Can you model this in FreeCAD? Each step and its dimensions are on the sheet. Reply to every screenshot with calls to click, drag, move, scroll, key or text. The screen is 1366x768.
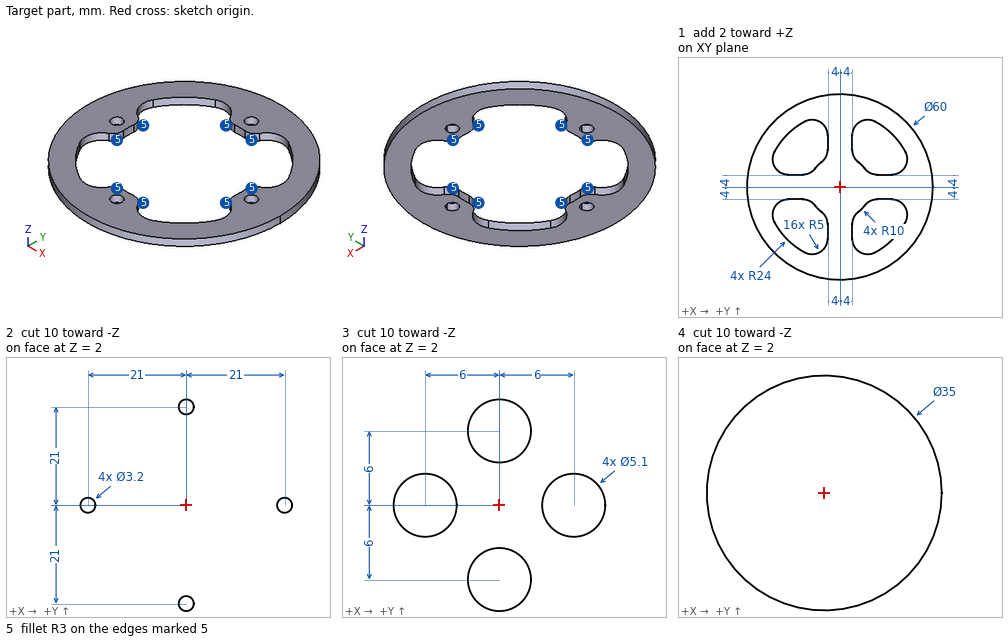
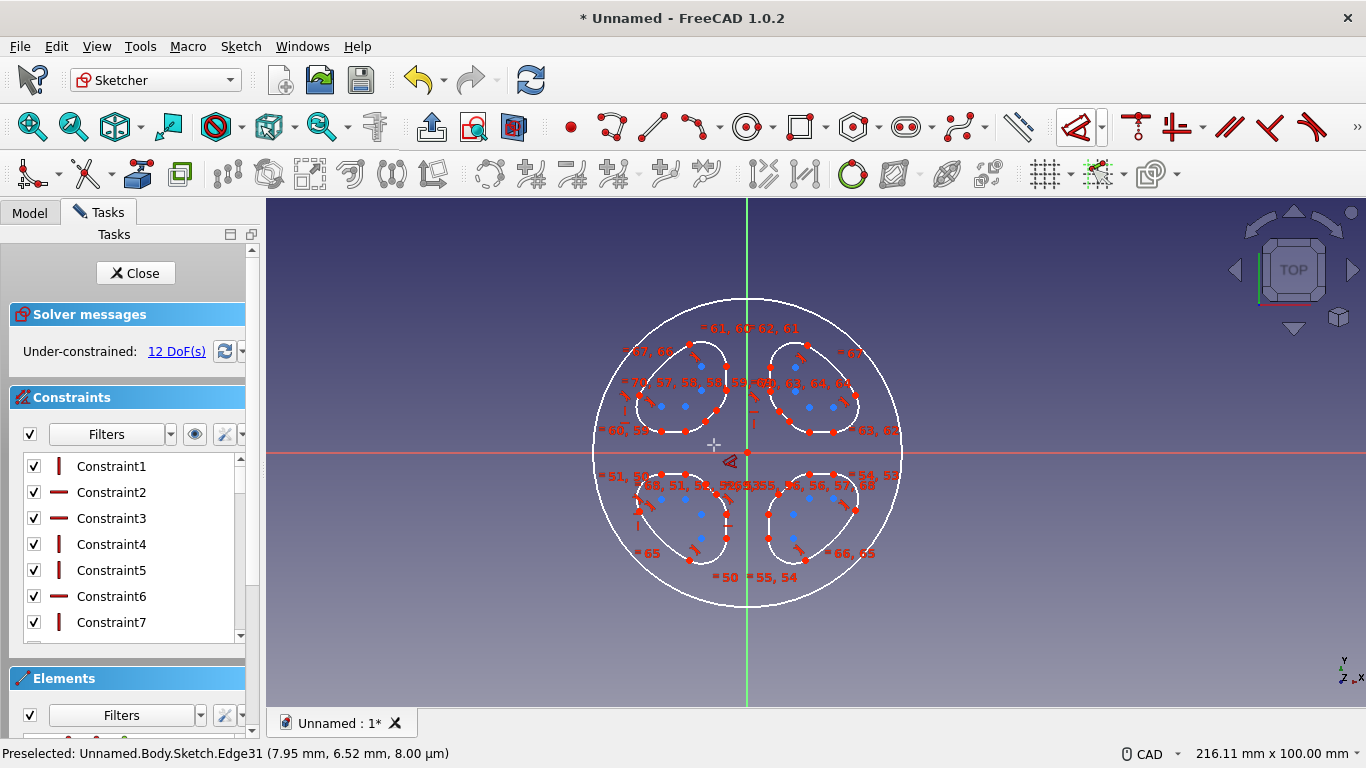
scroll(705, 563, up, 3)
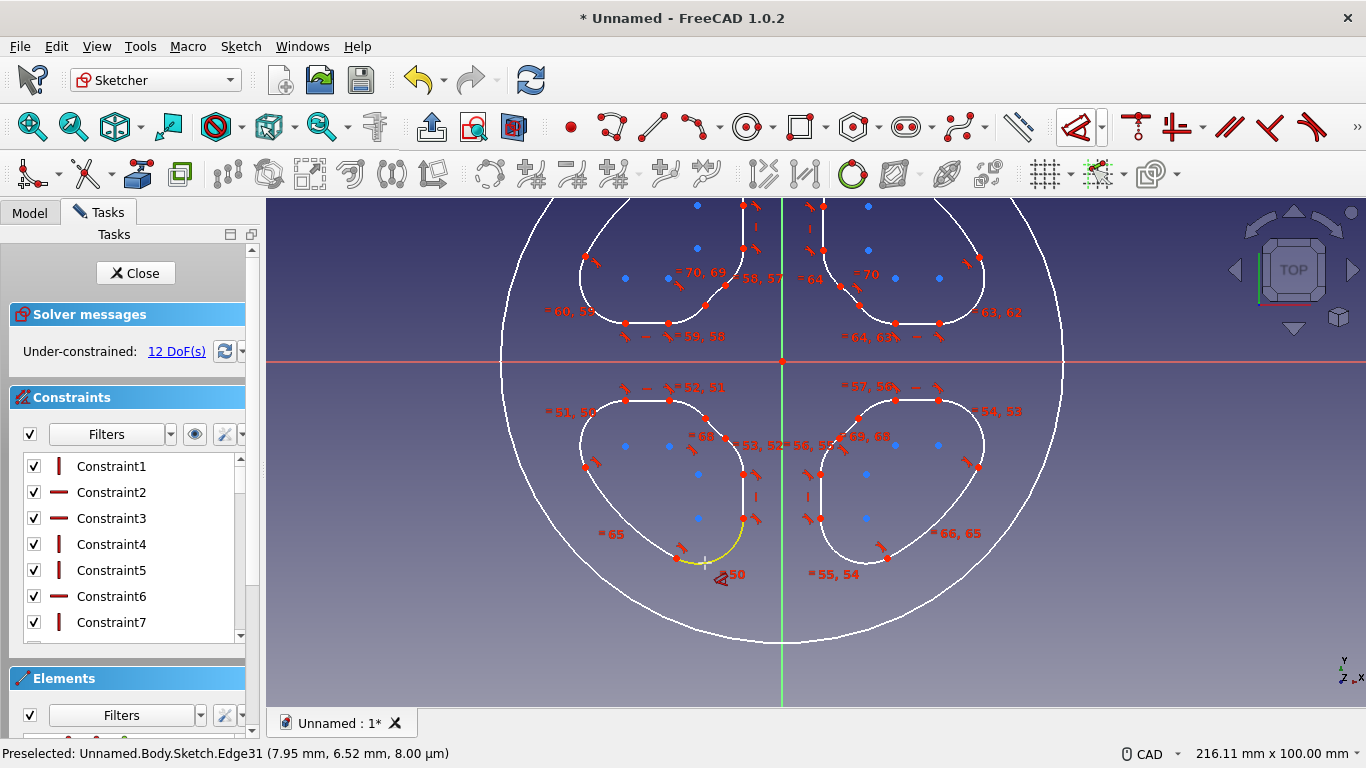
click(704, 563)
click(708, 595)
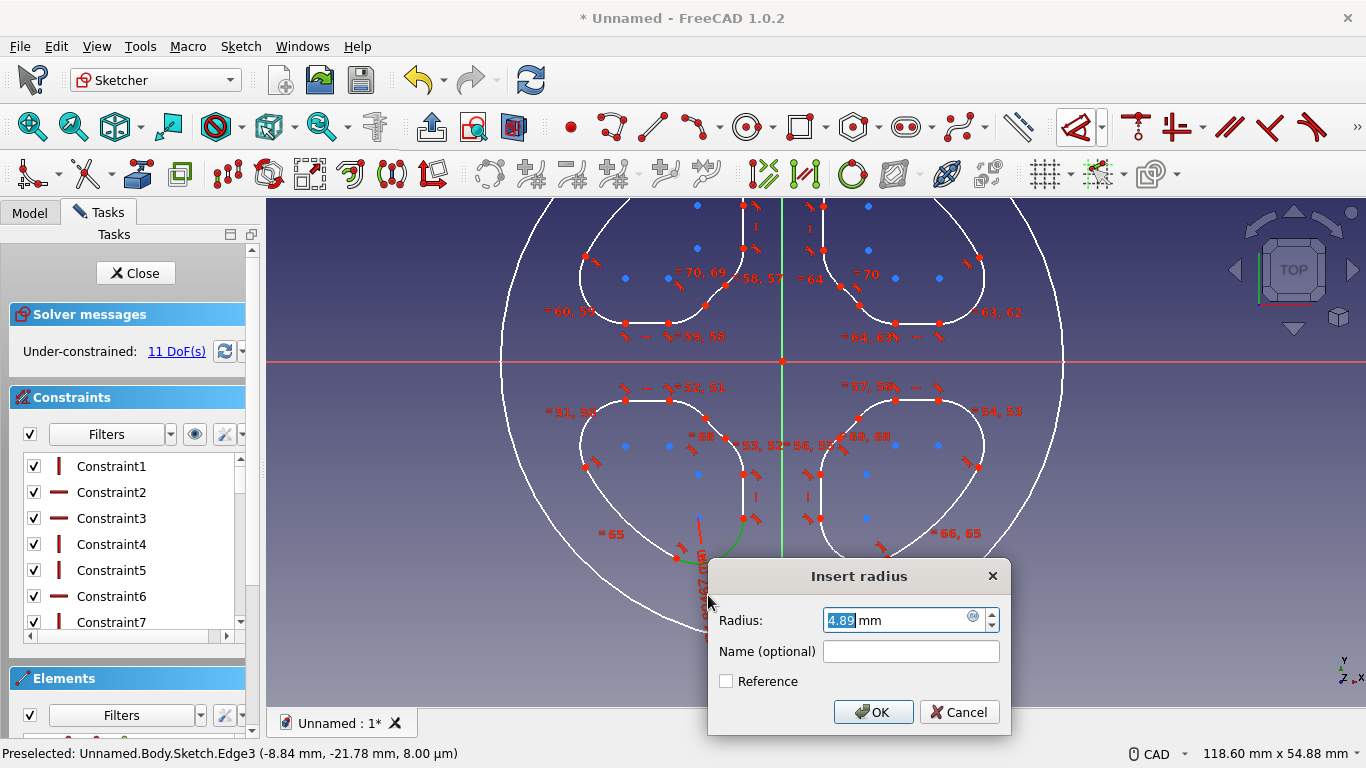
text(5)
key(Return)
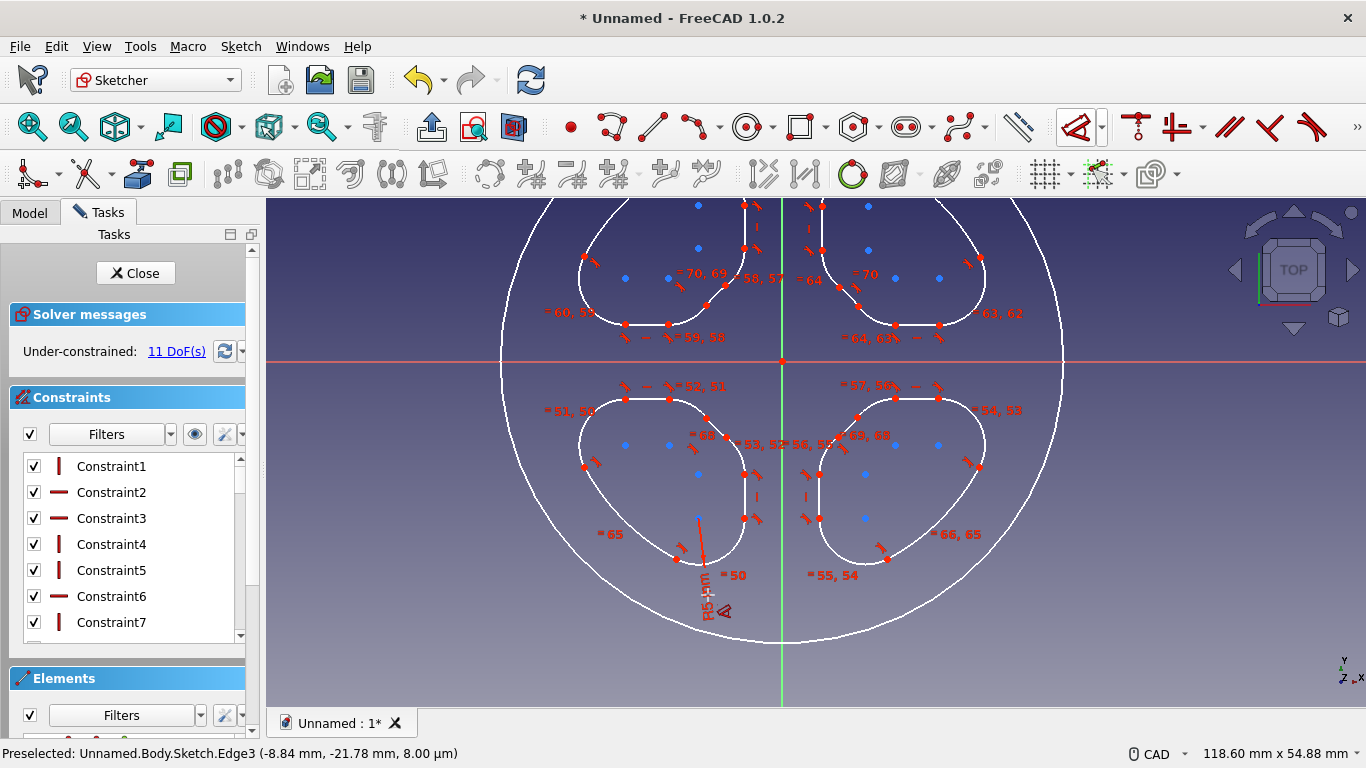
click(607, 501)
click(582, 521)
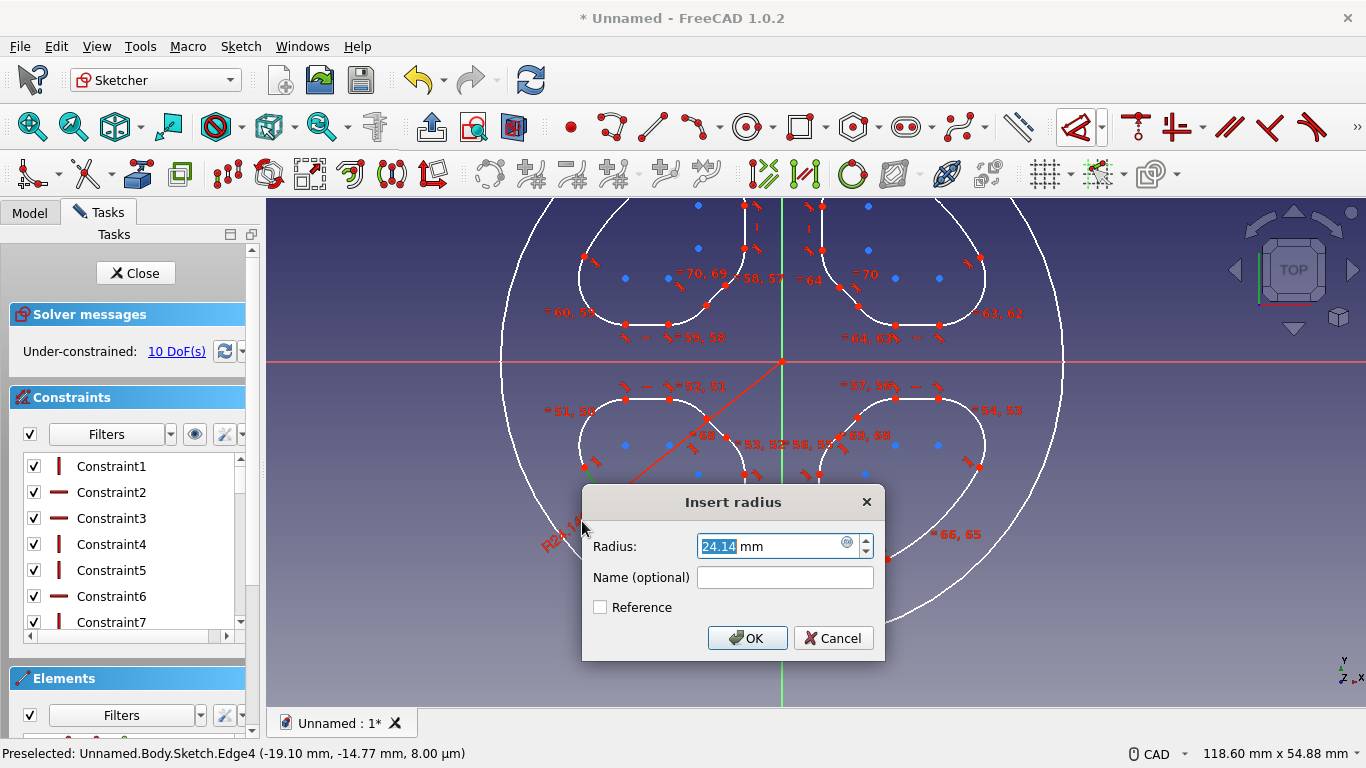
text(24)
key(Return)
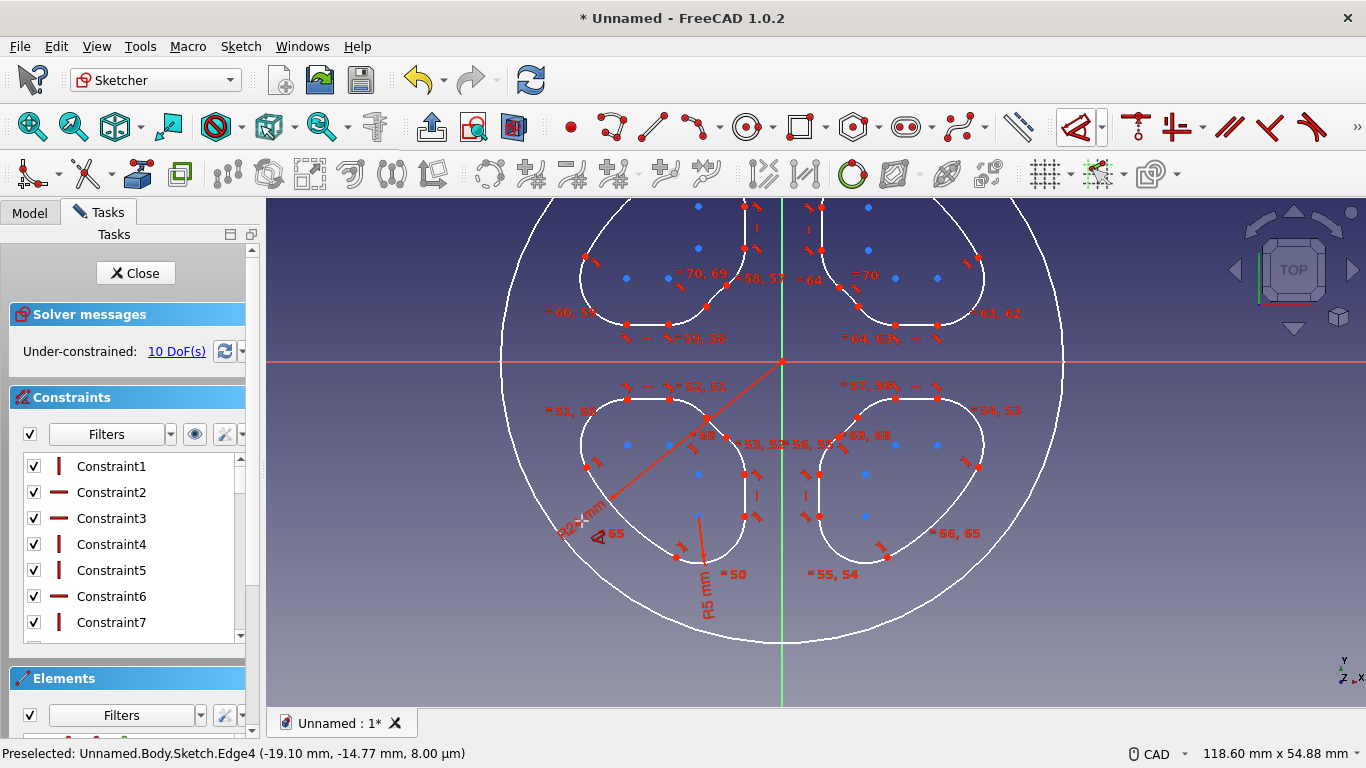
click(716, 428)
click(693, 451)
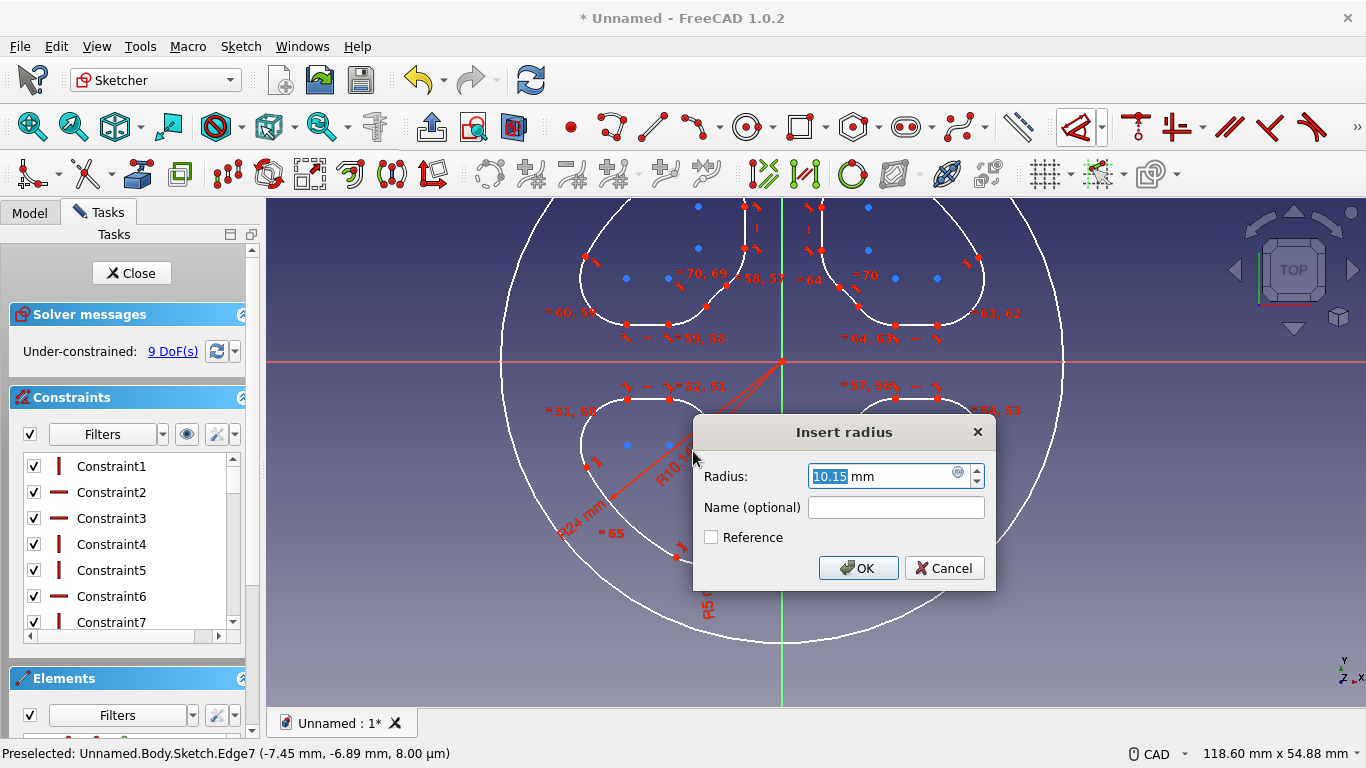
text(10)
key(Return)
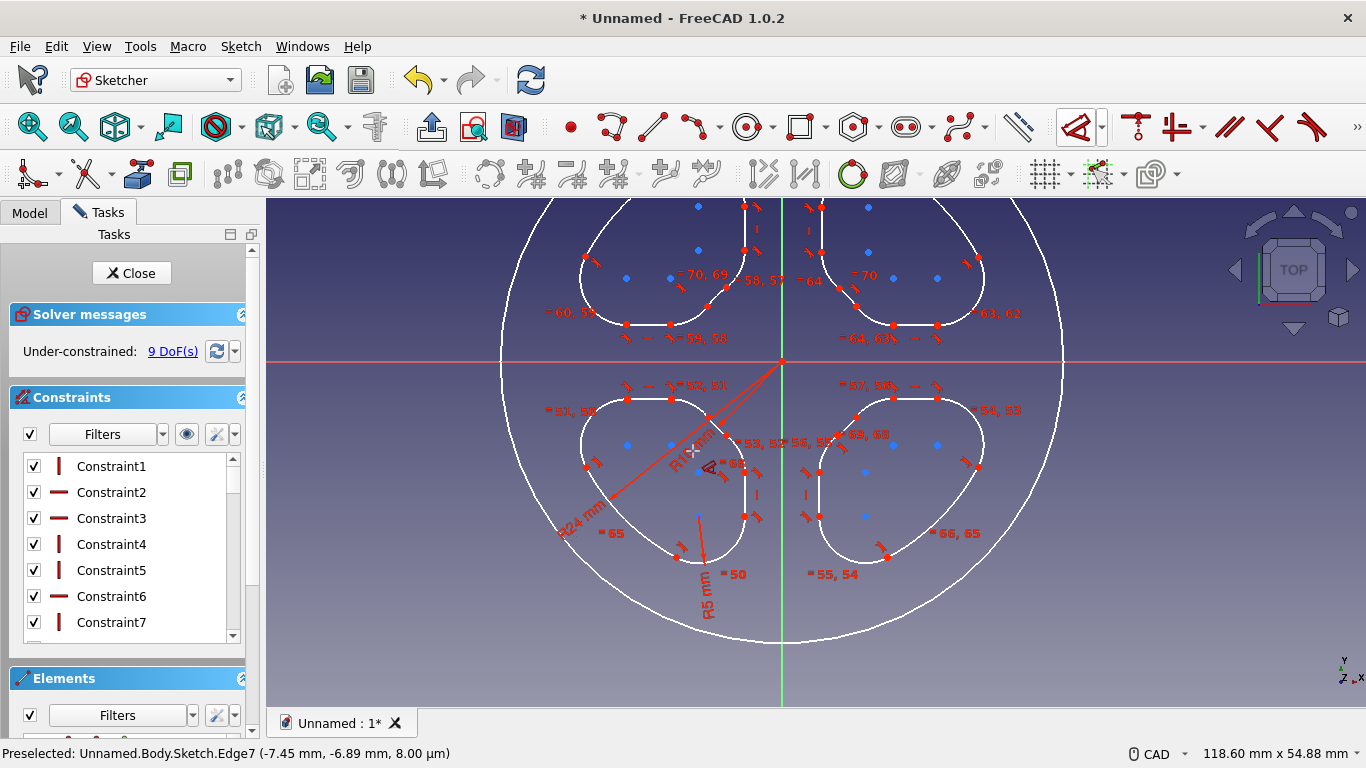
click(584, 561)
click(561, 584)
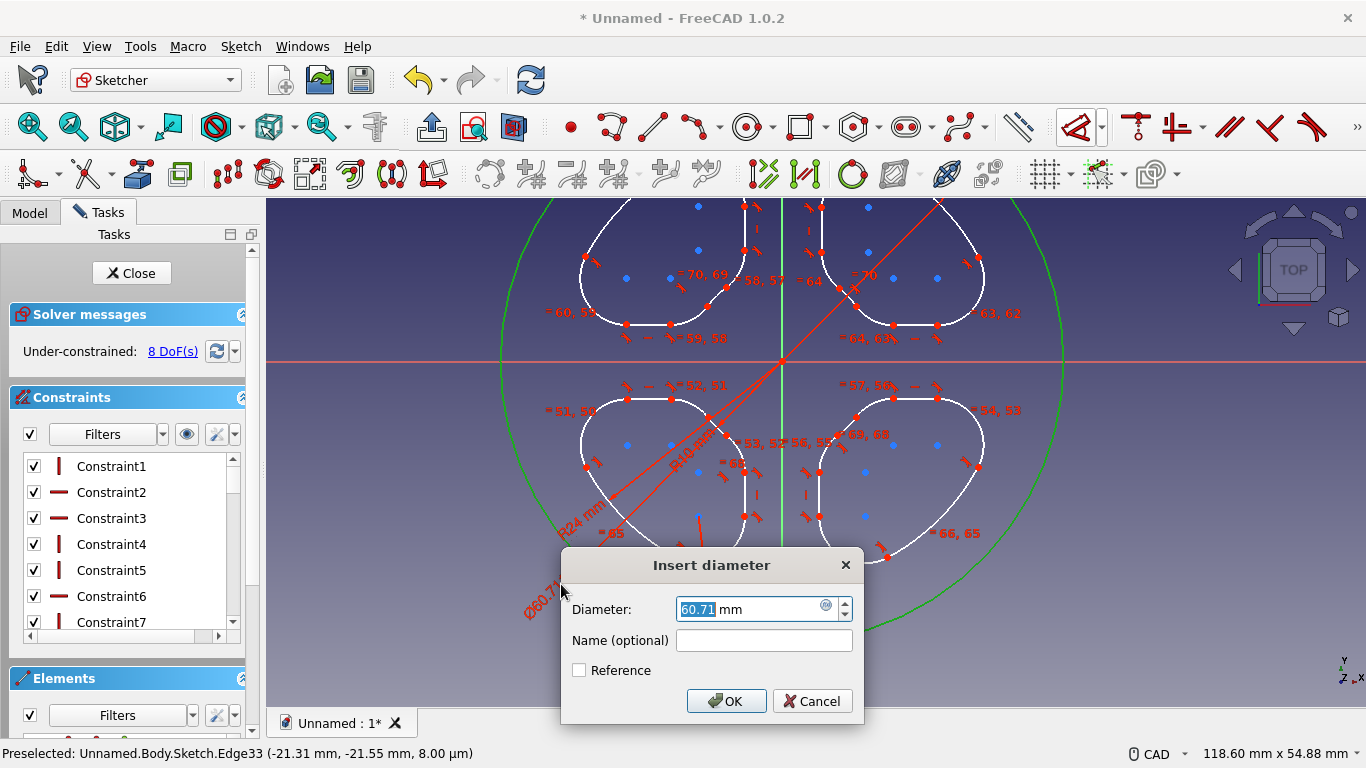
text(60)
key(Return)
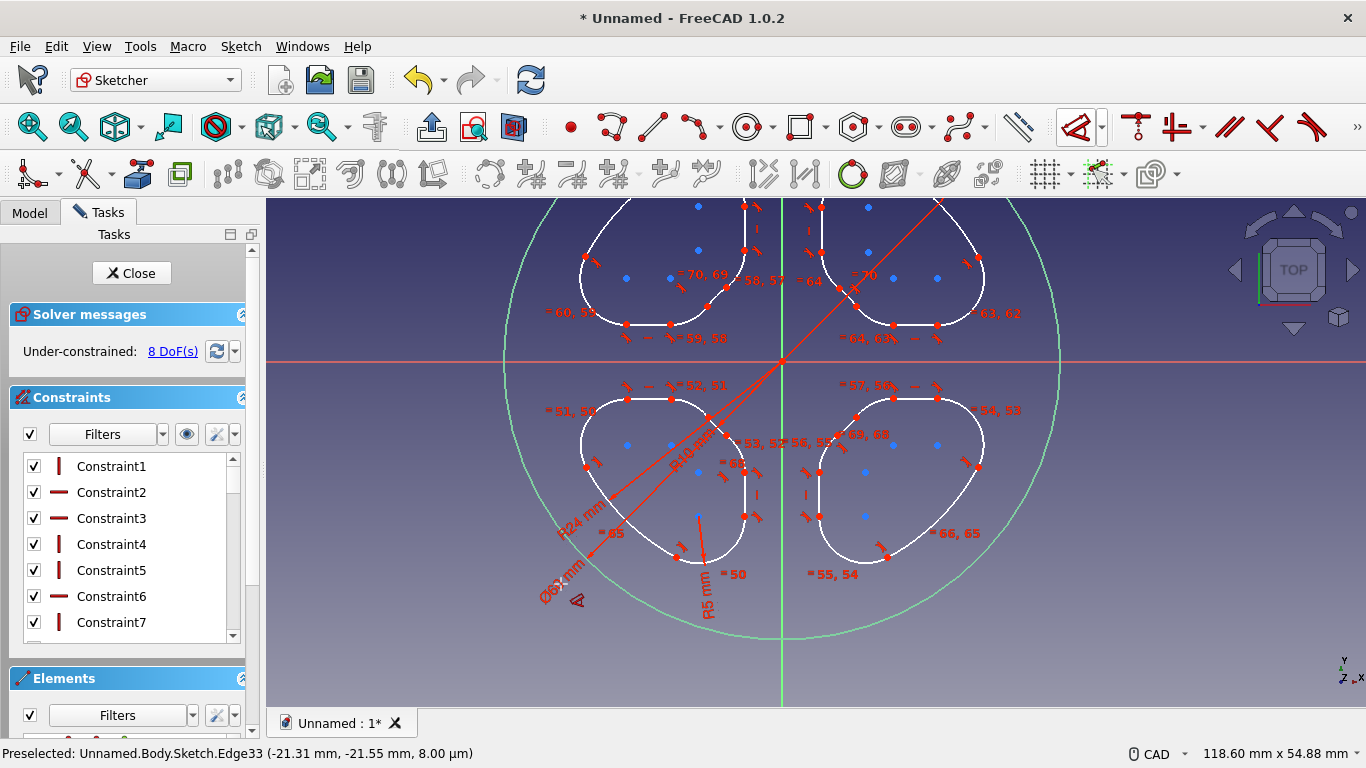
click(745, 473)
click(763, 507)